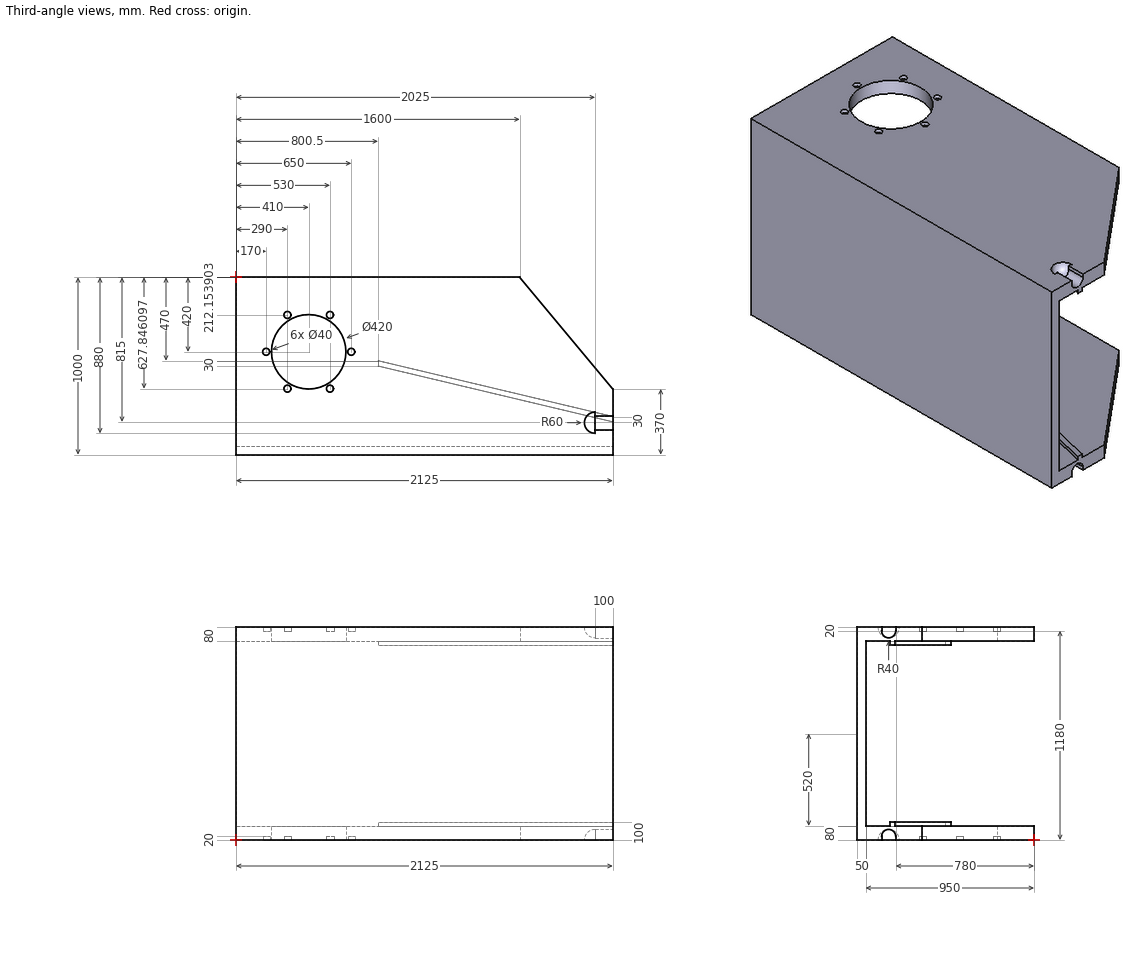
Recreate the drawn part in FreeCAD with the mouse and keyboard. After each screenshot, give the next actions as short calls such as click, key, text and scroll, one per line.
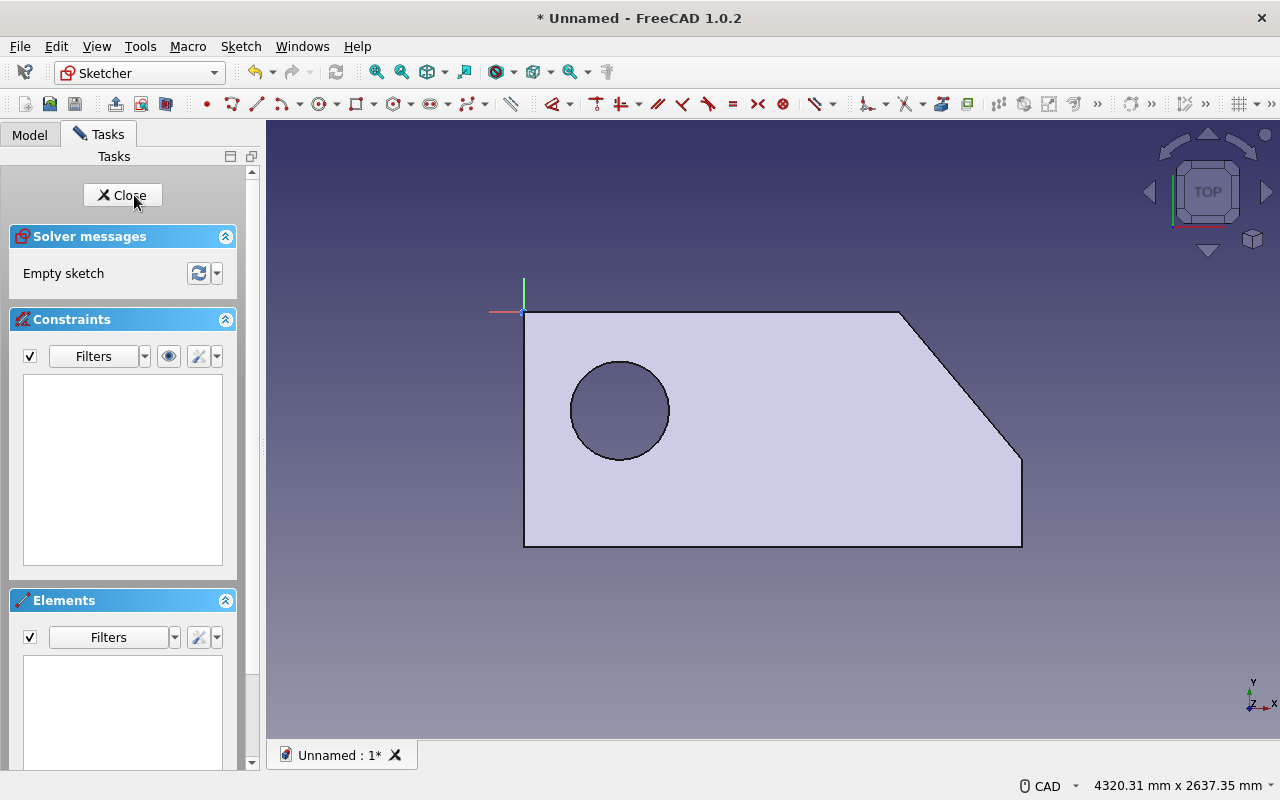
key(q)
key(s)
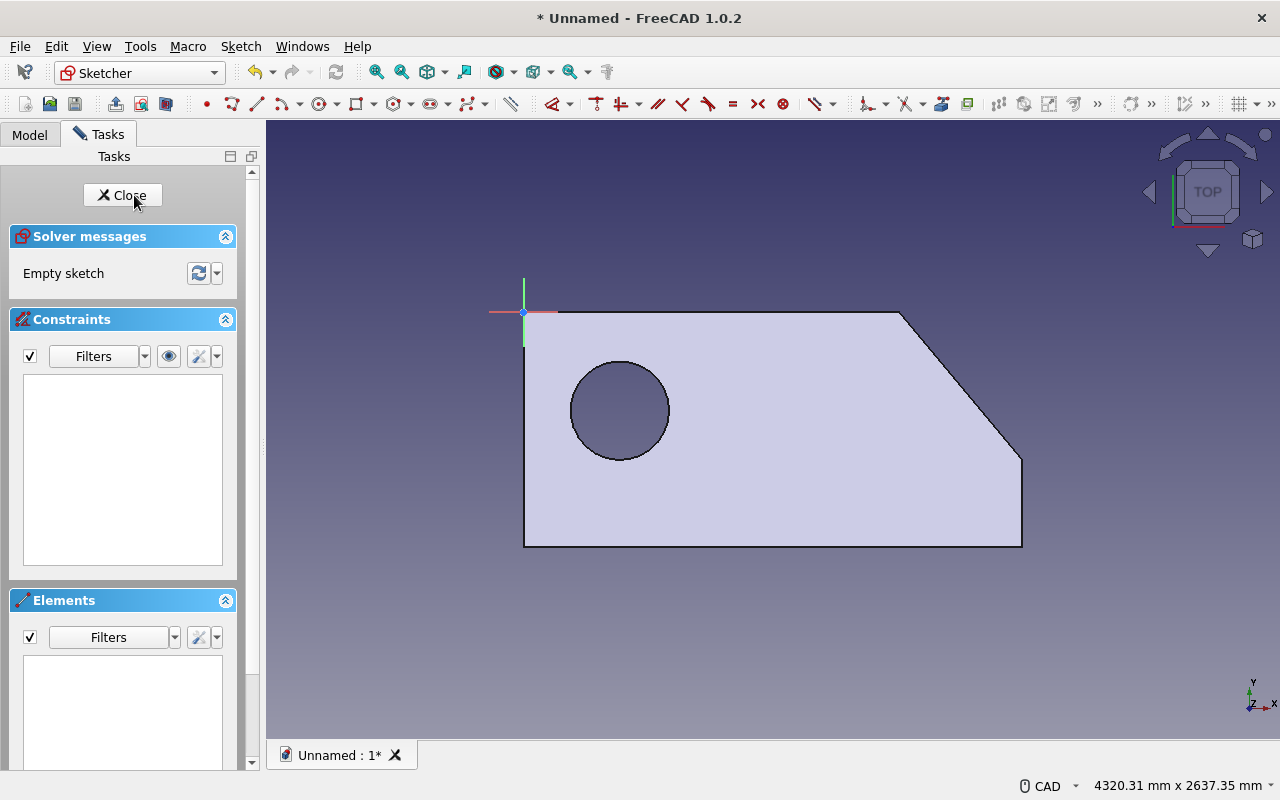
key(g)
key(m)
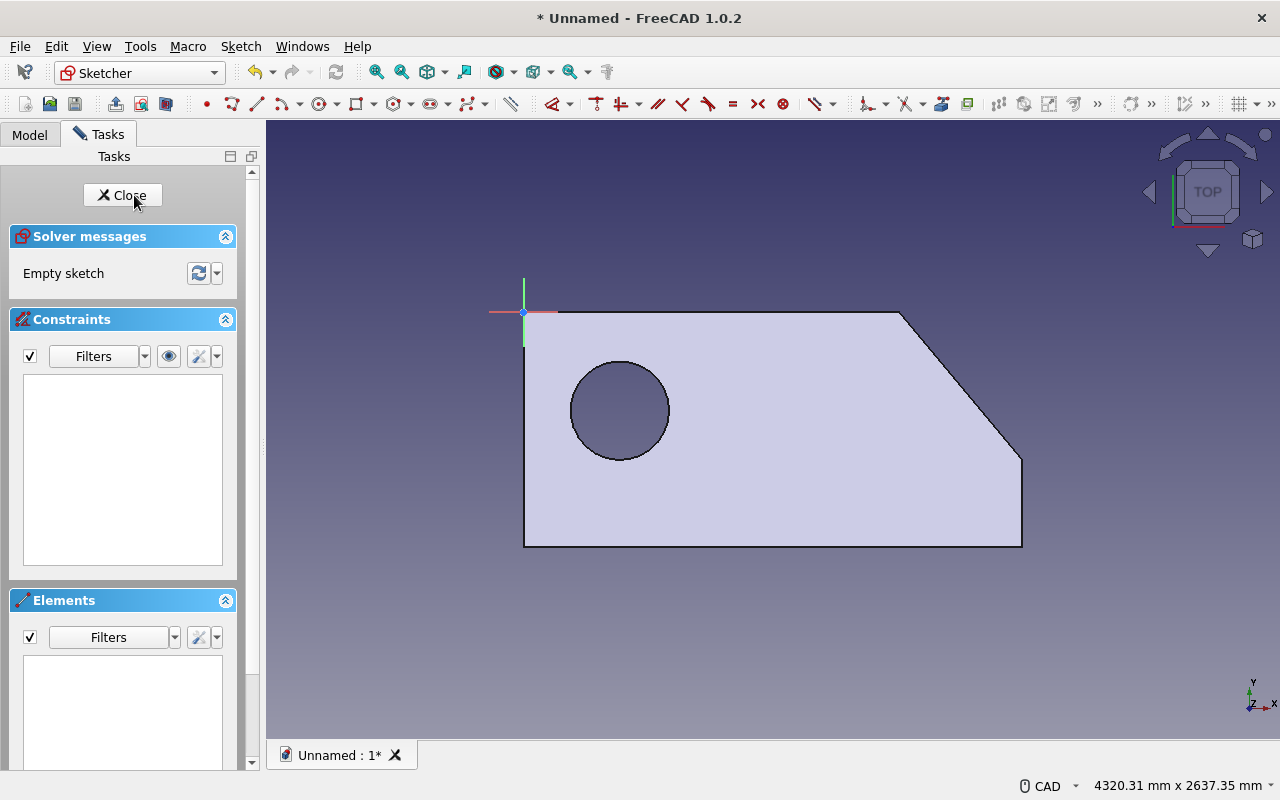
click(712, 422)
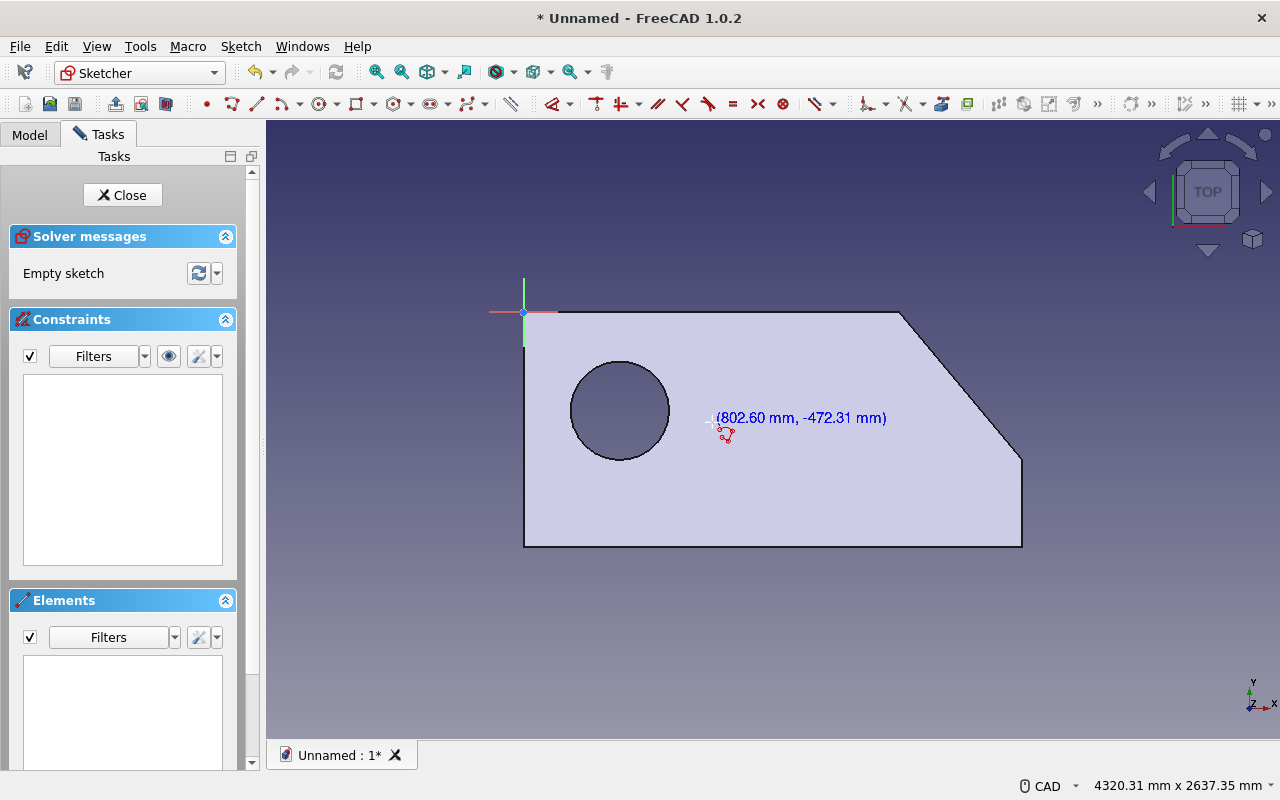
scroll(712, 429, up, 5)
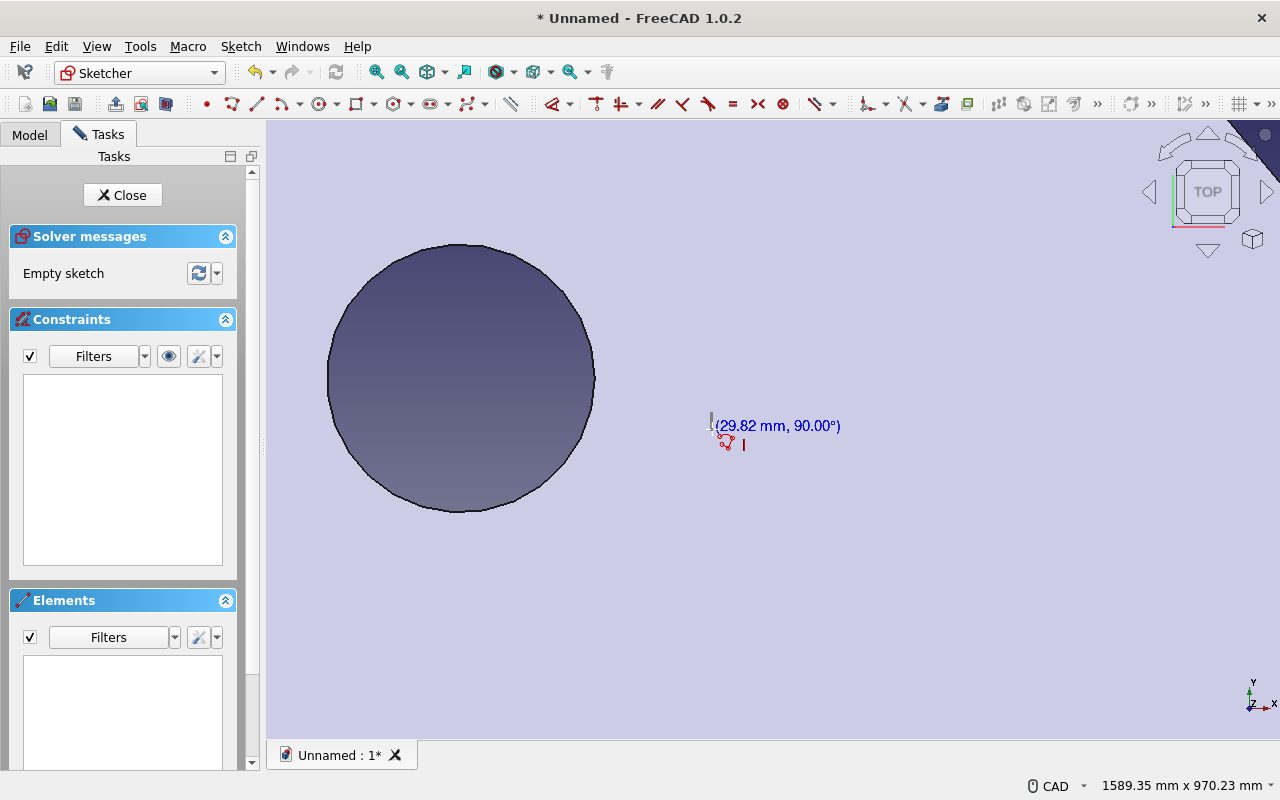
click(711, 429)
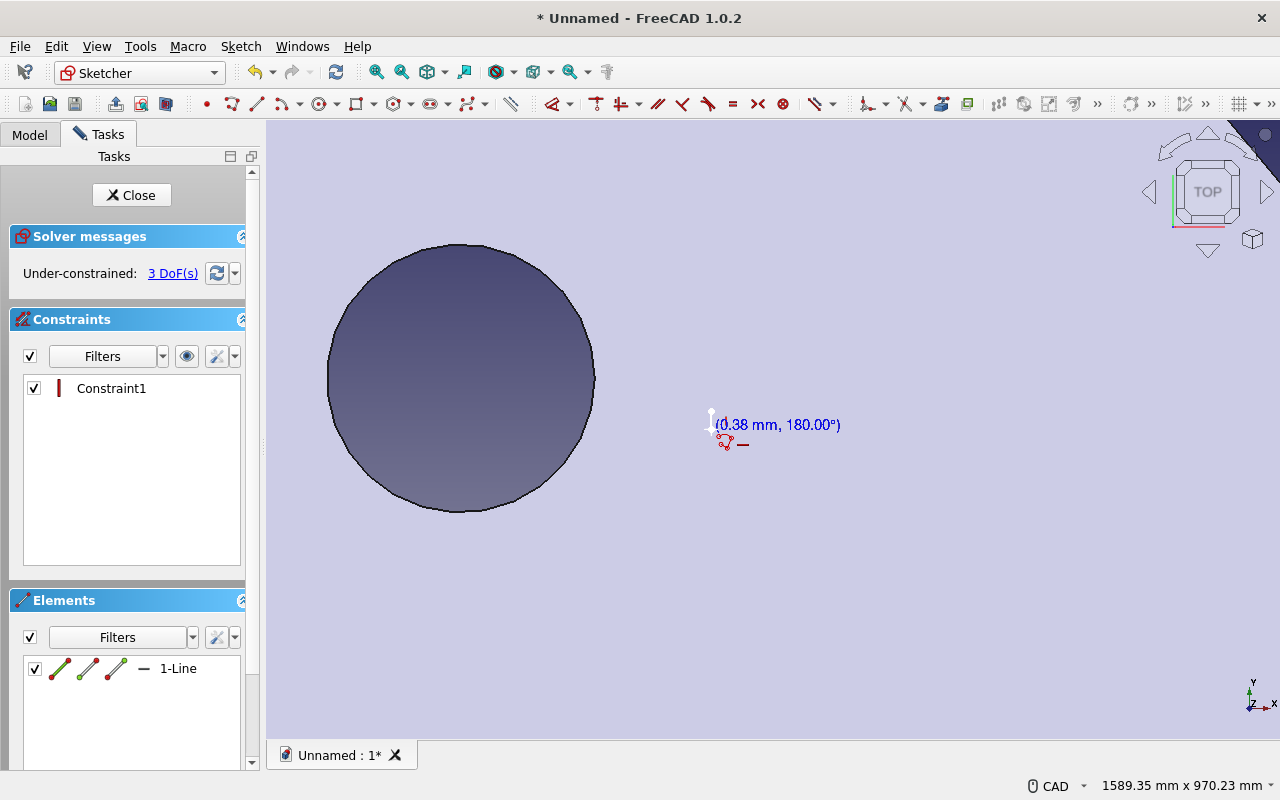
scroll(564, 478, down, 4)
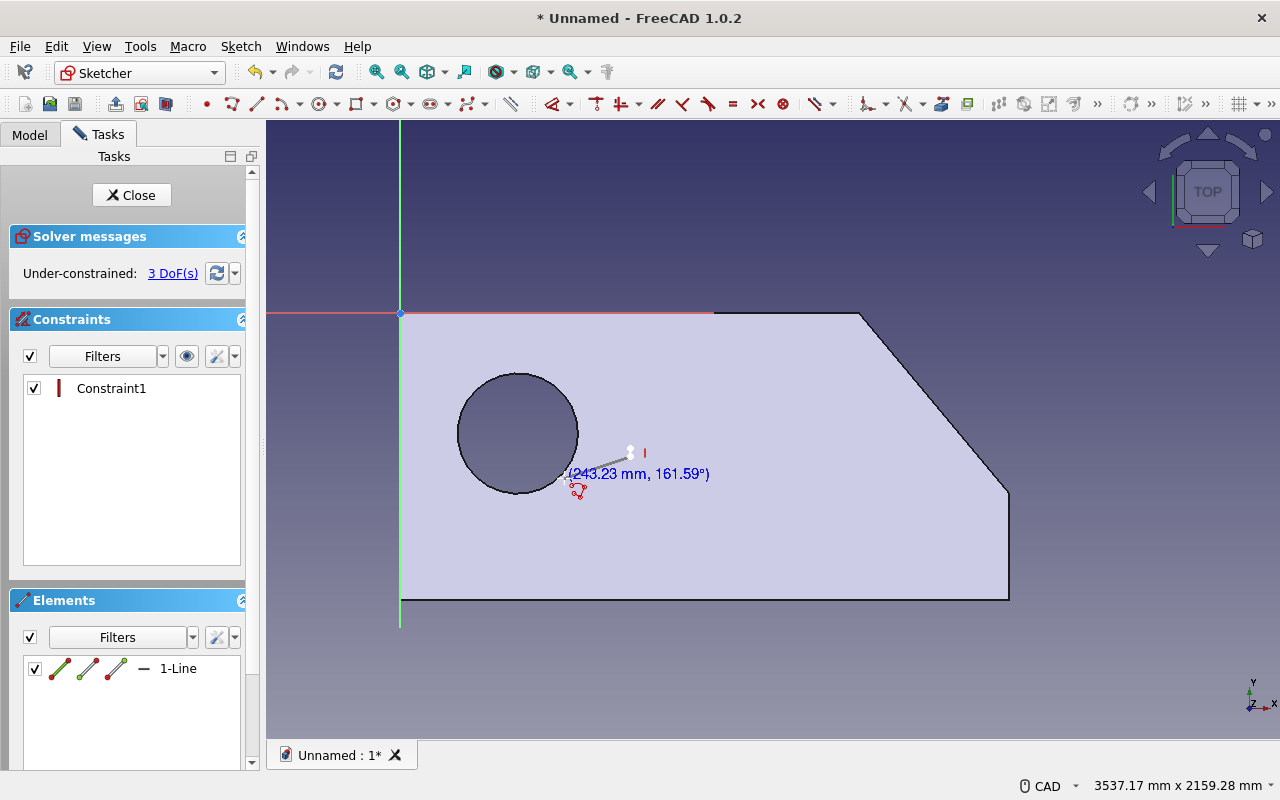
click(1009, 547)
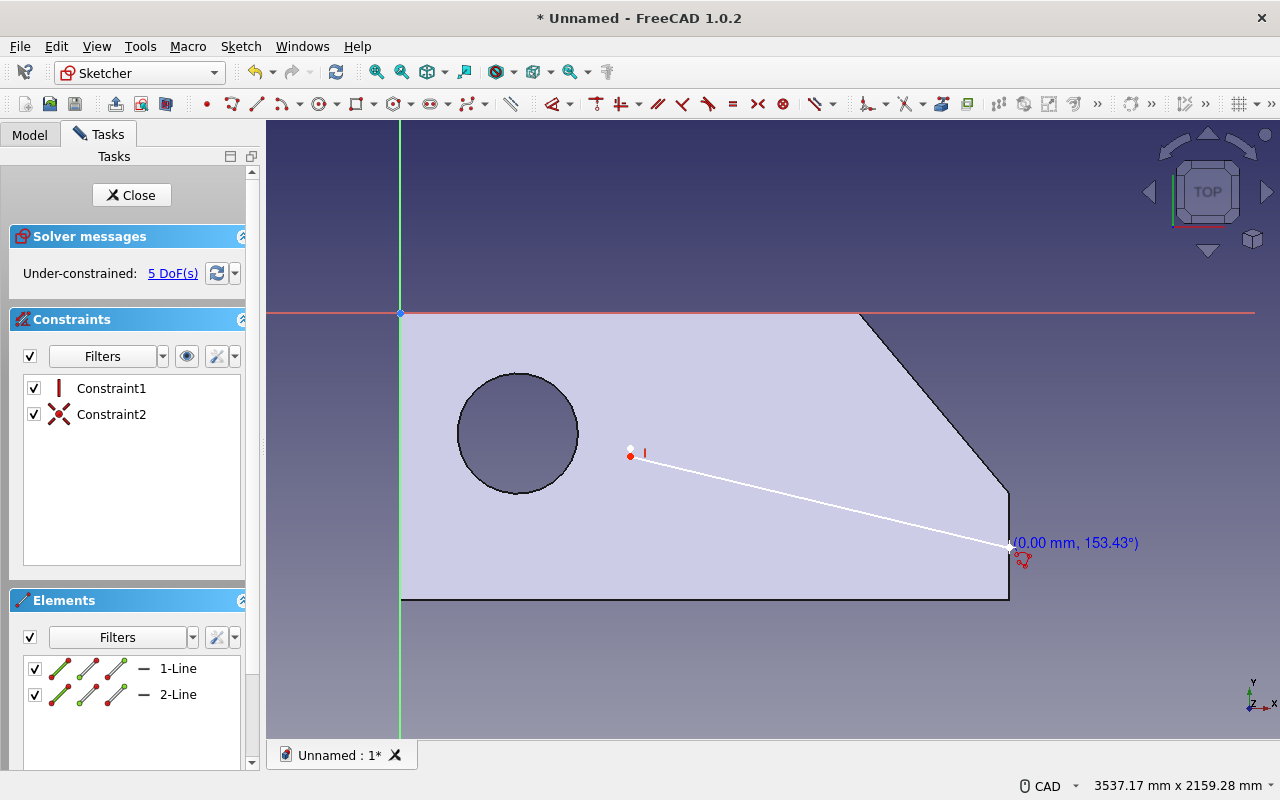
scroll(1009, 538, up, 4)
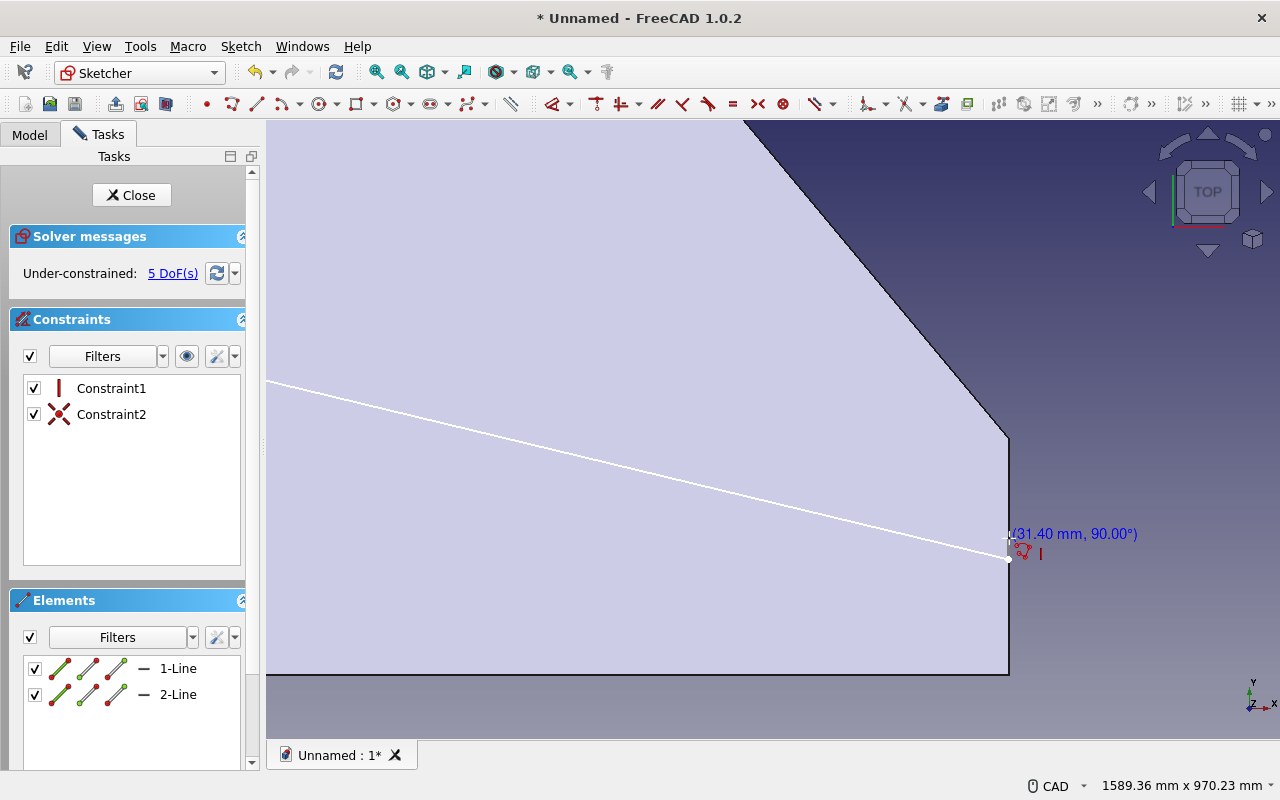
click(1008, 538)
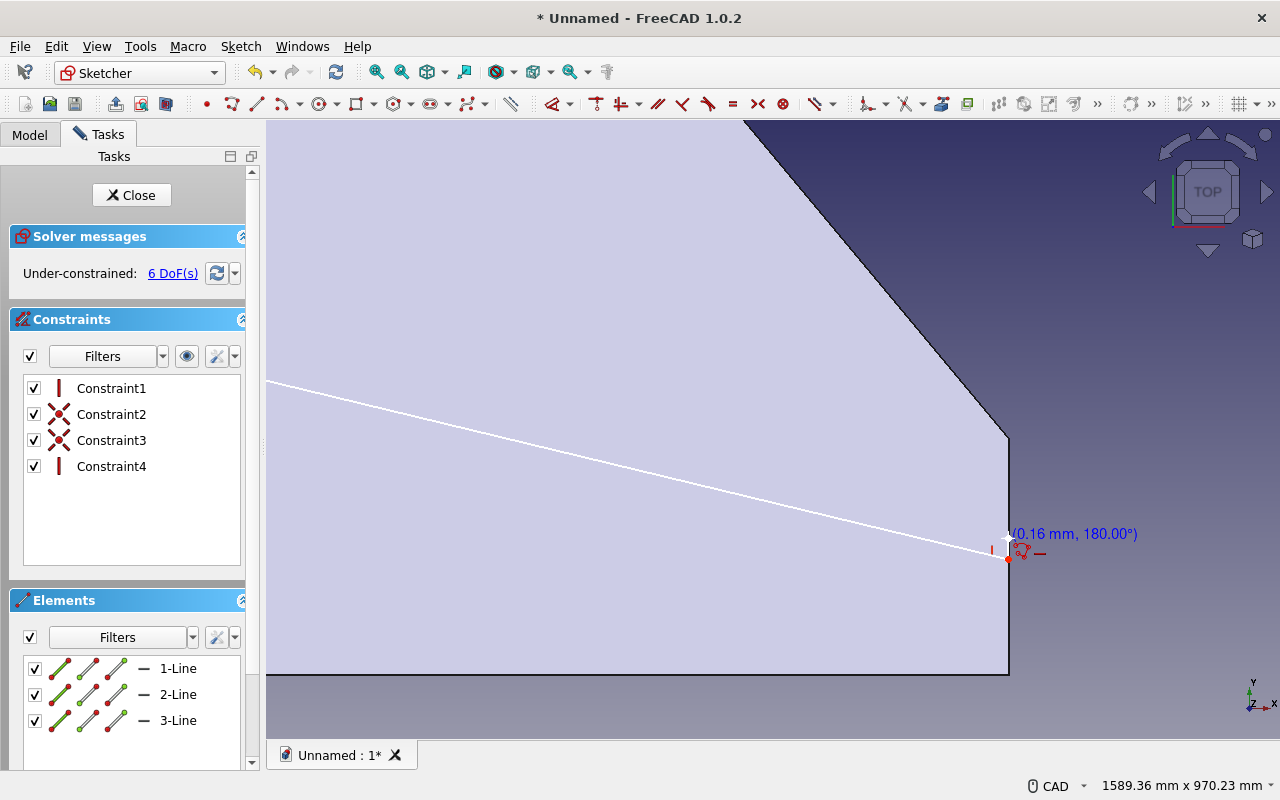
scroll(1009, 538, down, 4)